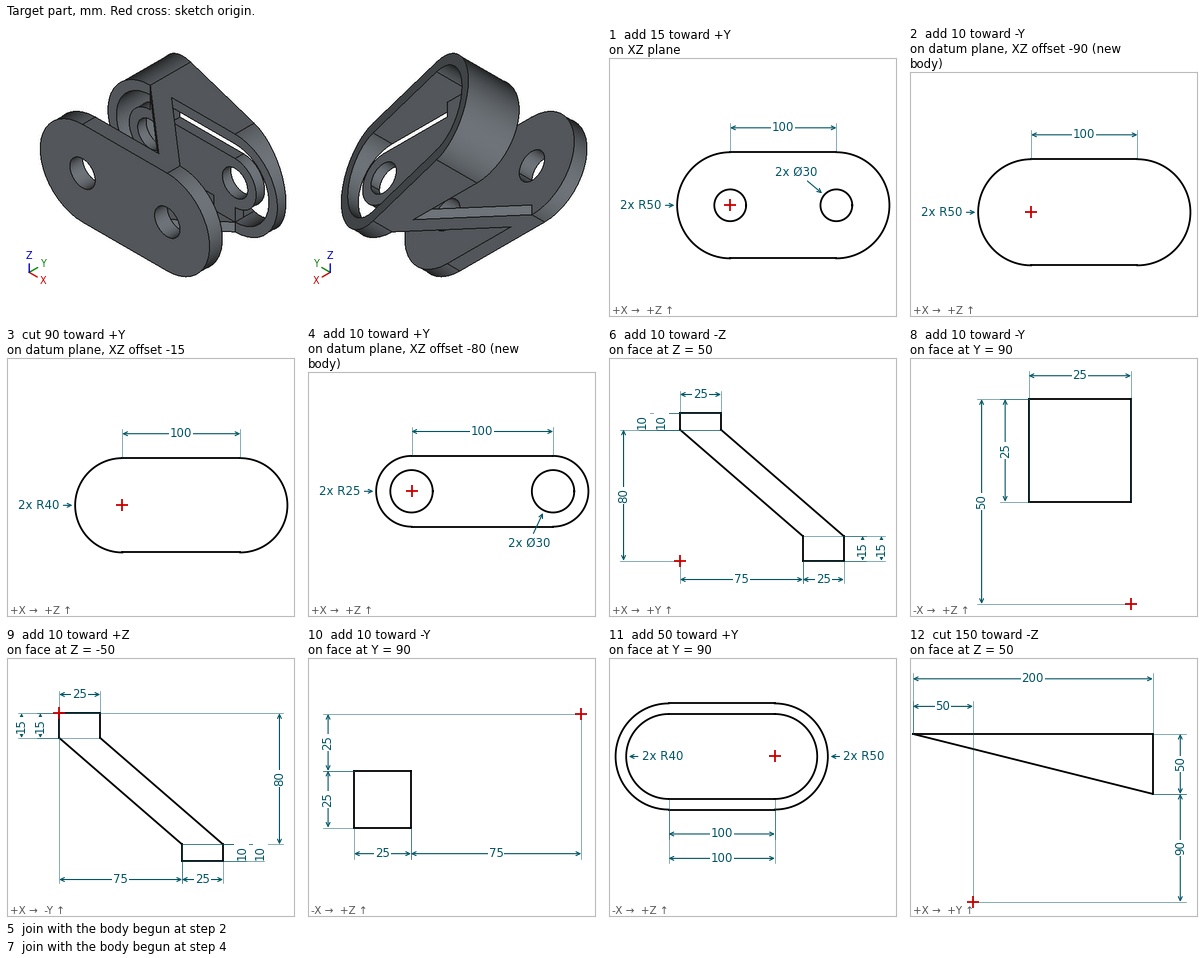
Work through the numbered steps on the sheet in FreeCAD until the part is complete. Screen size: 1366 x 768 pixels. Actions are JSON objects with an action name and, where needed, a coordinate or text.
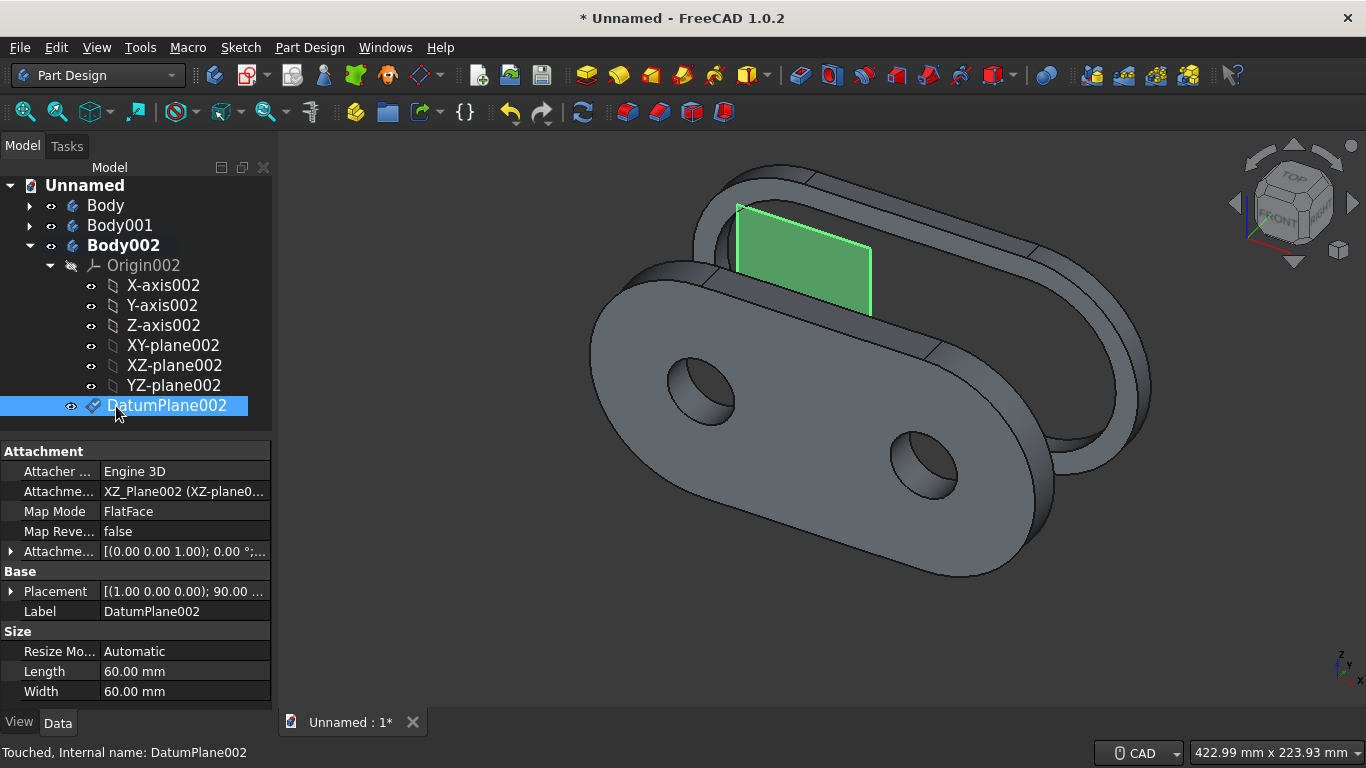
{"action": "left_click", "coordinate": [248, 76]}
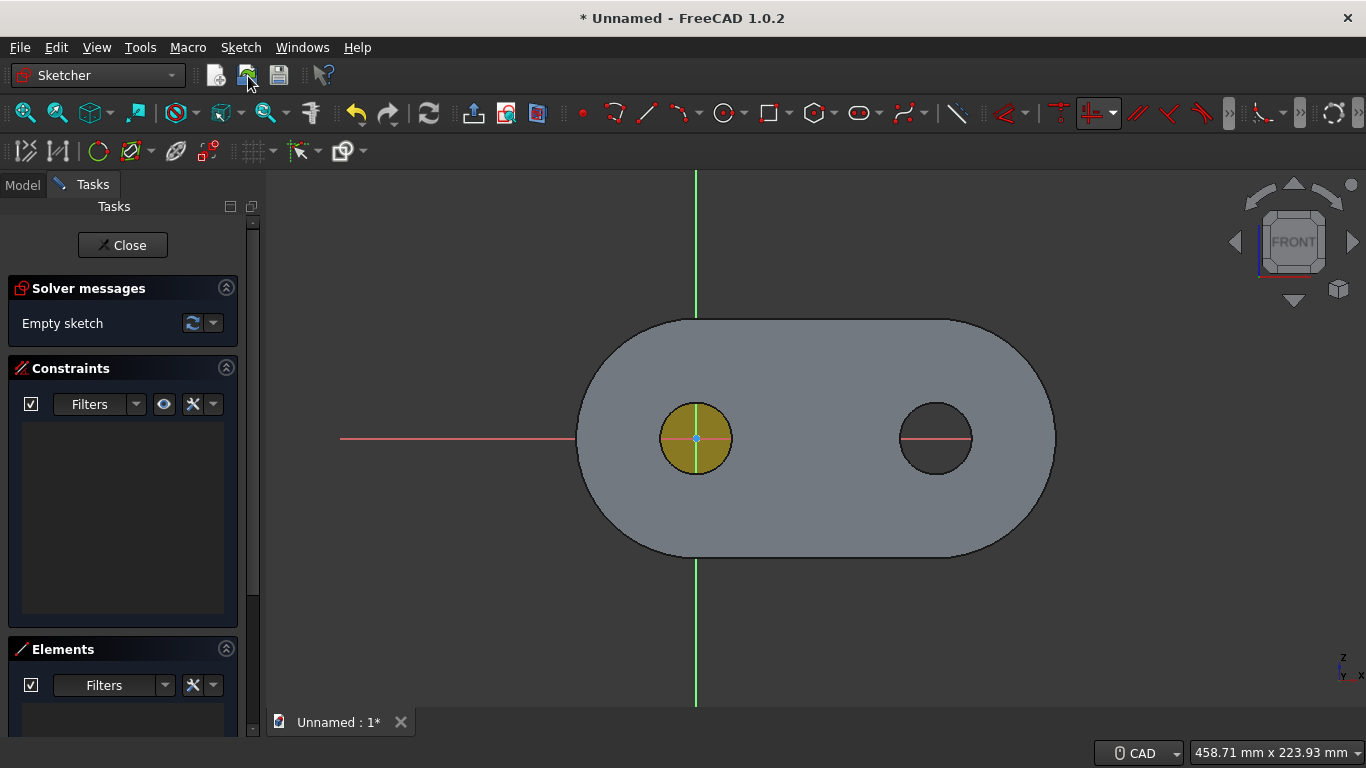
{"action": "scroll", "coordinate": [899, 439], "scroll_direction": "up", "scroll_amount": 3}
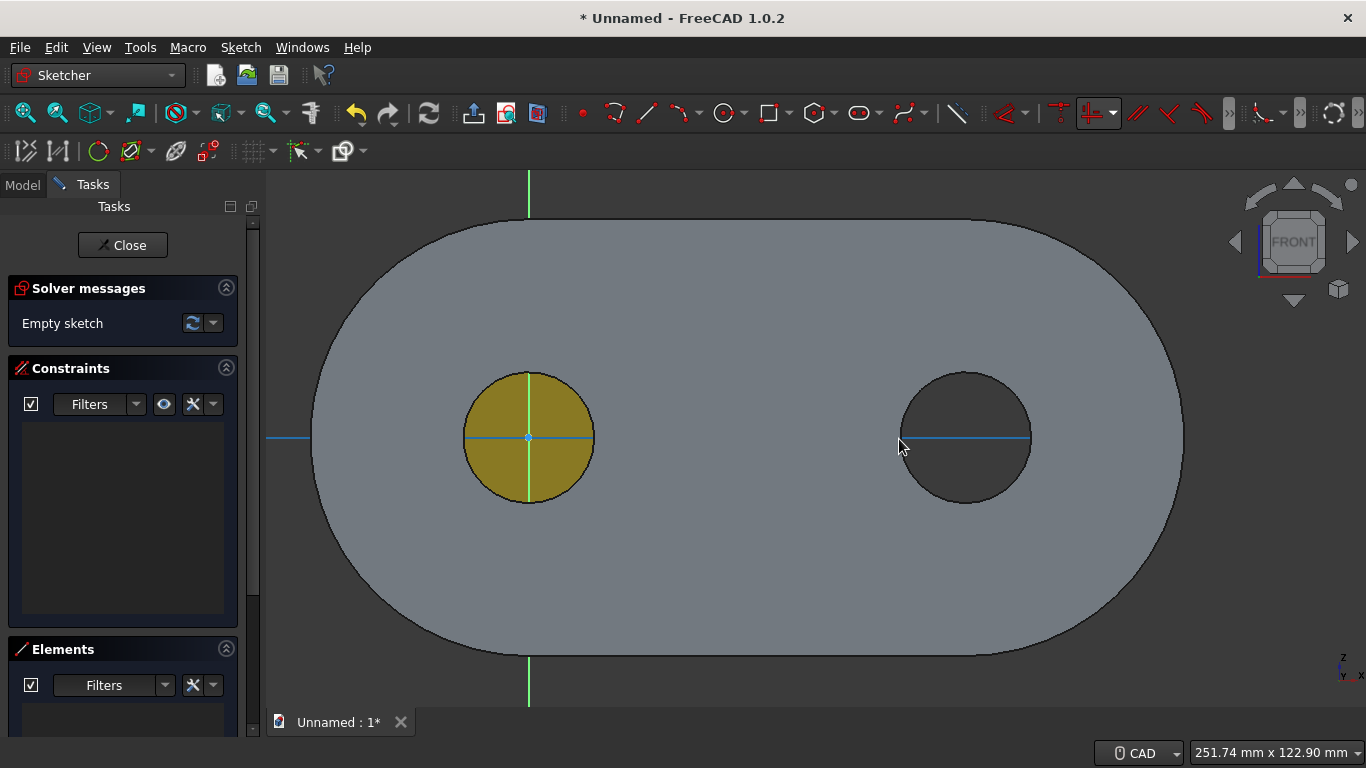
{"action": "left_click", "coordinate": [860, 114]}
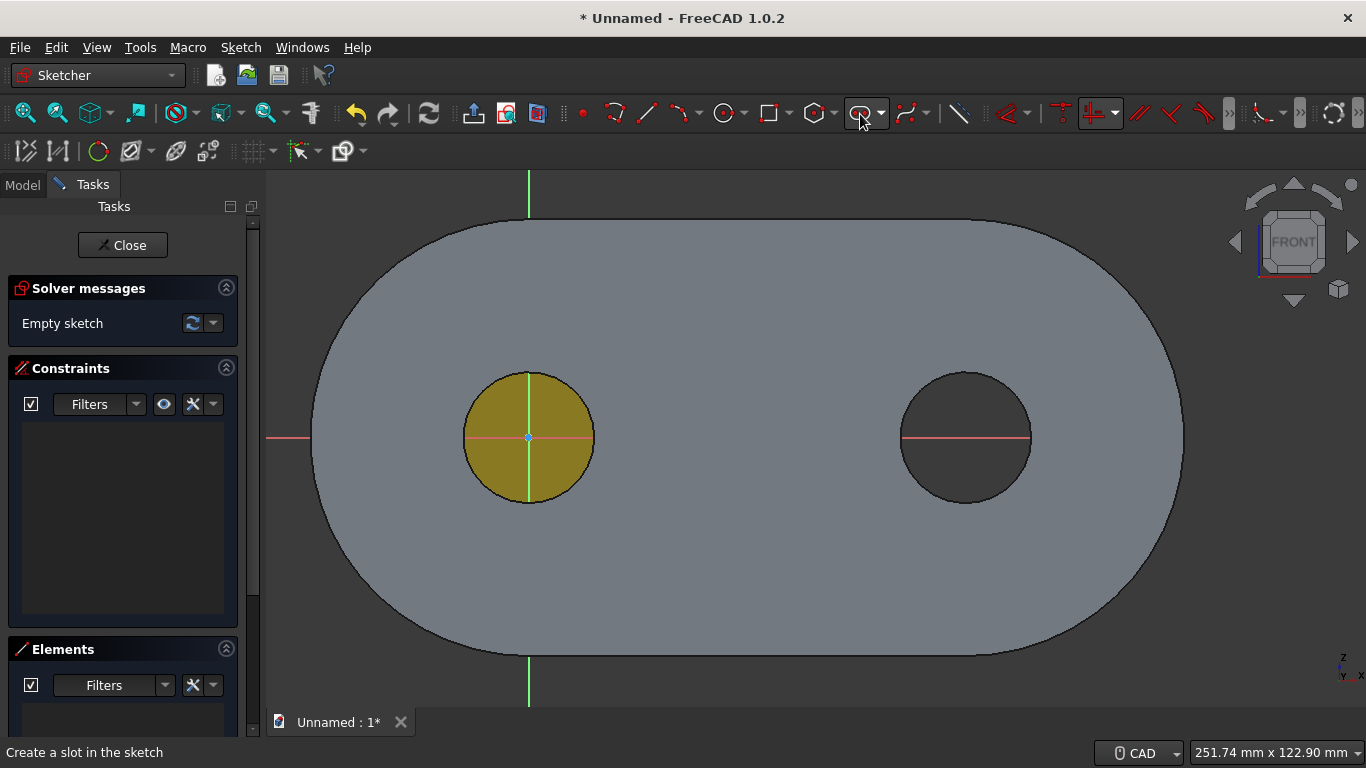
{"action": "left_click", "coordinate": [529, 438]}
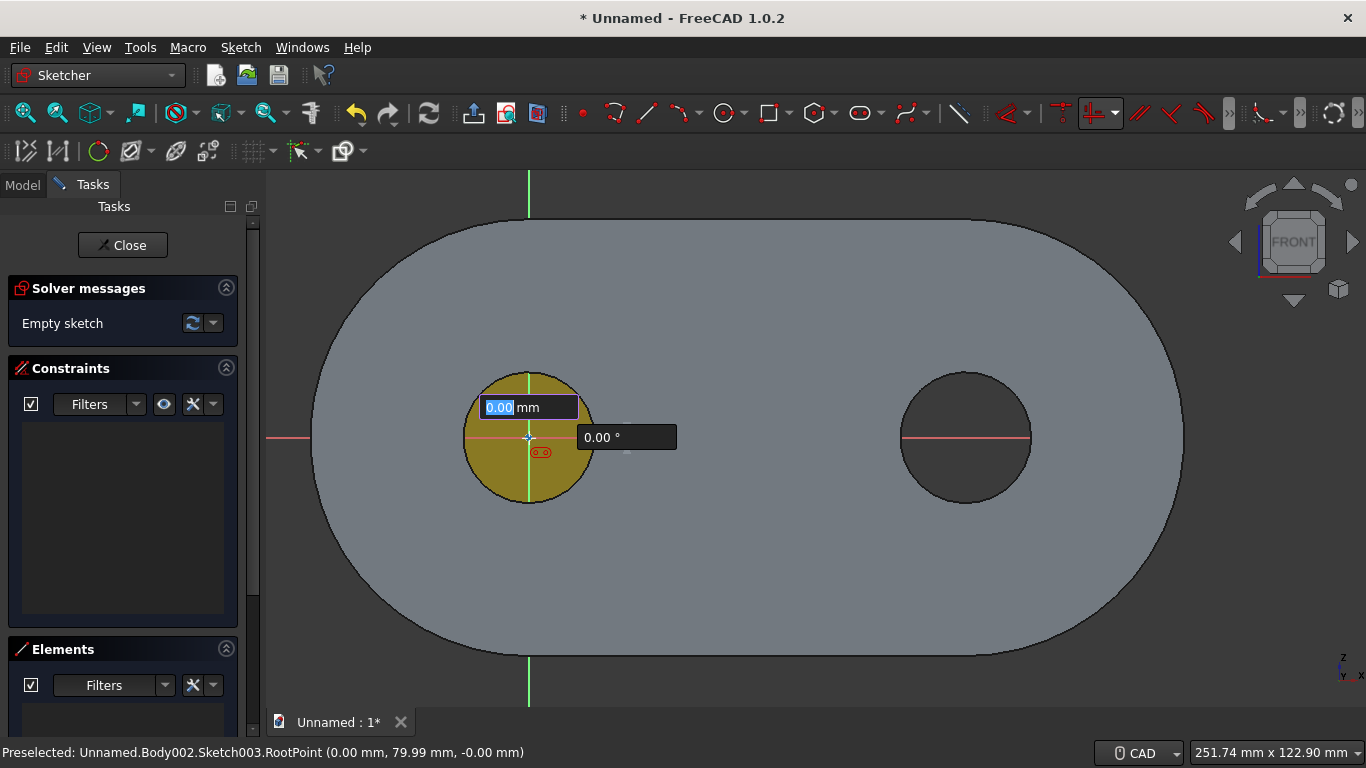
{"action": "left_click", "coordinate": [966, 429]}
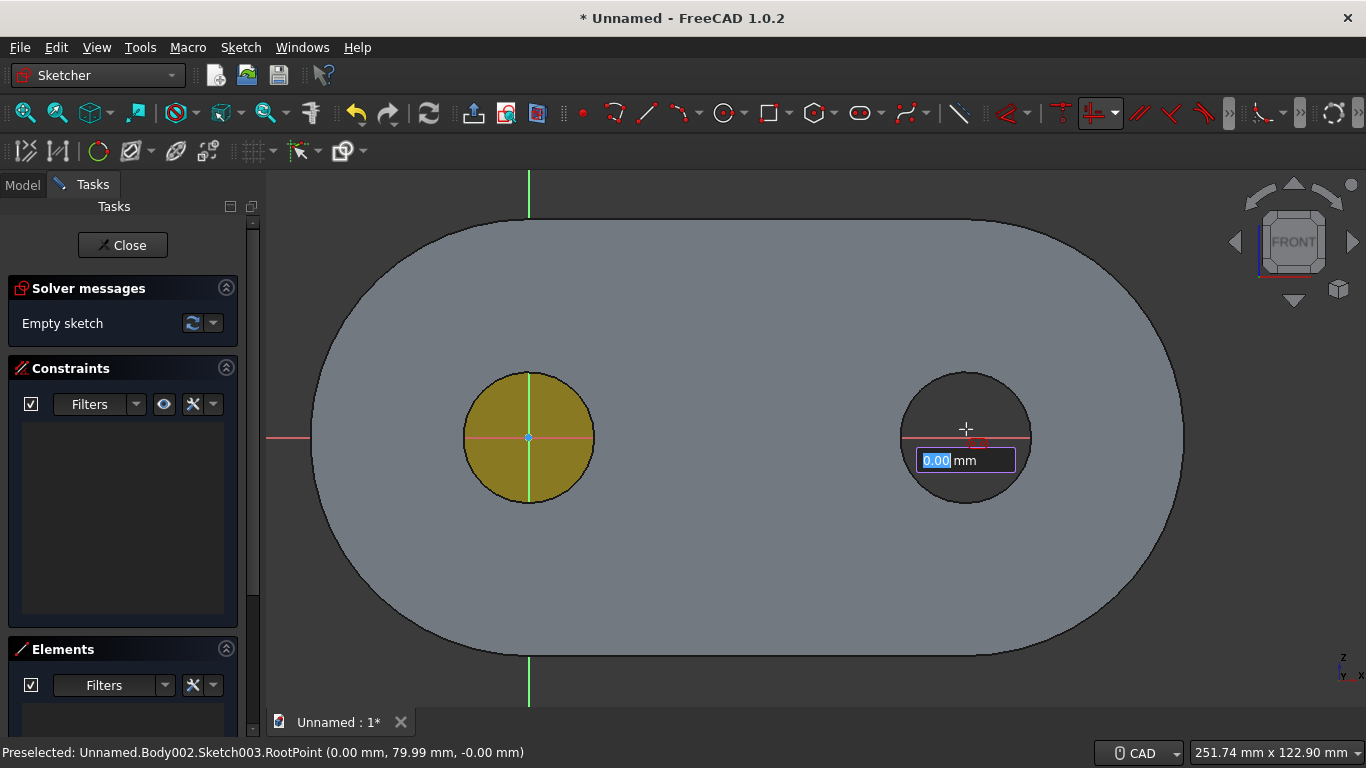
{"action": "left_click", "coordinate": [747, 547]}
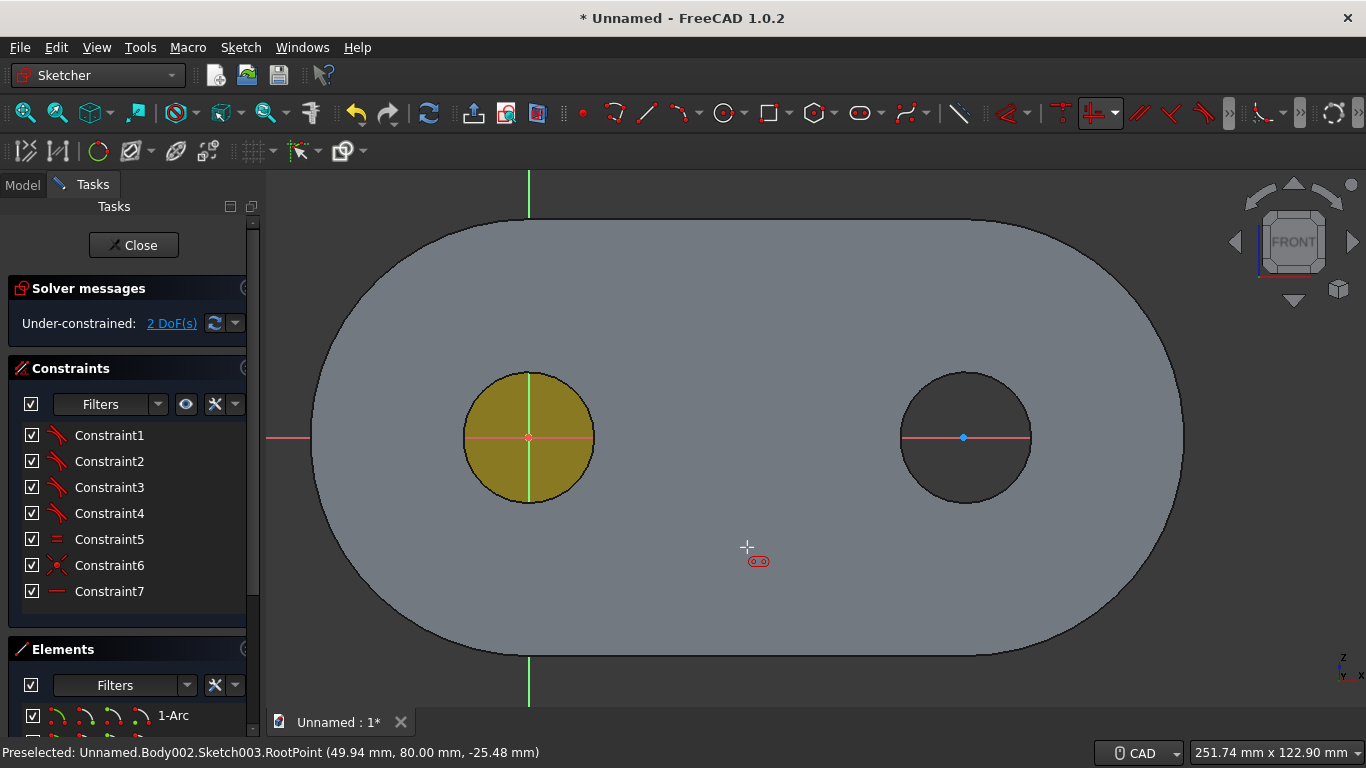
{"action": "left_click", "coordinate": [724, 114]}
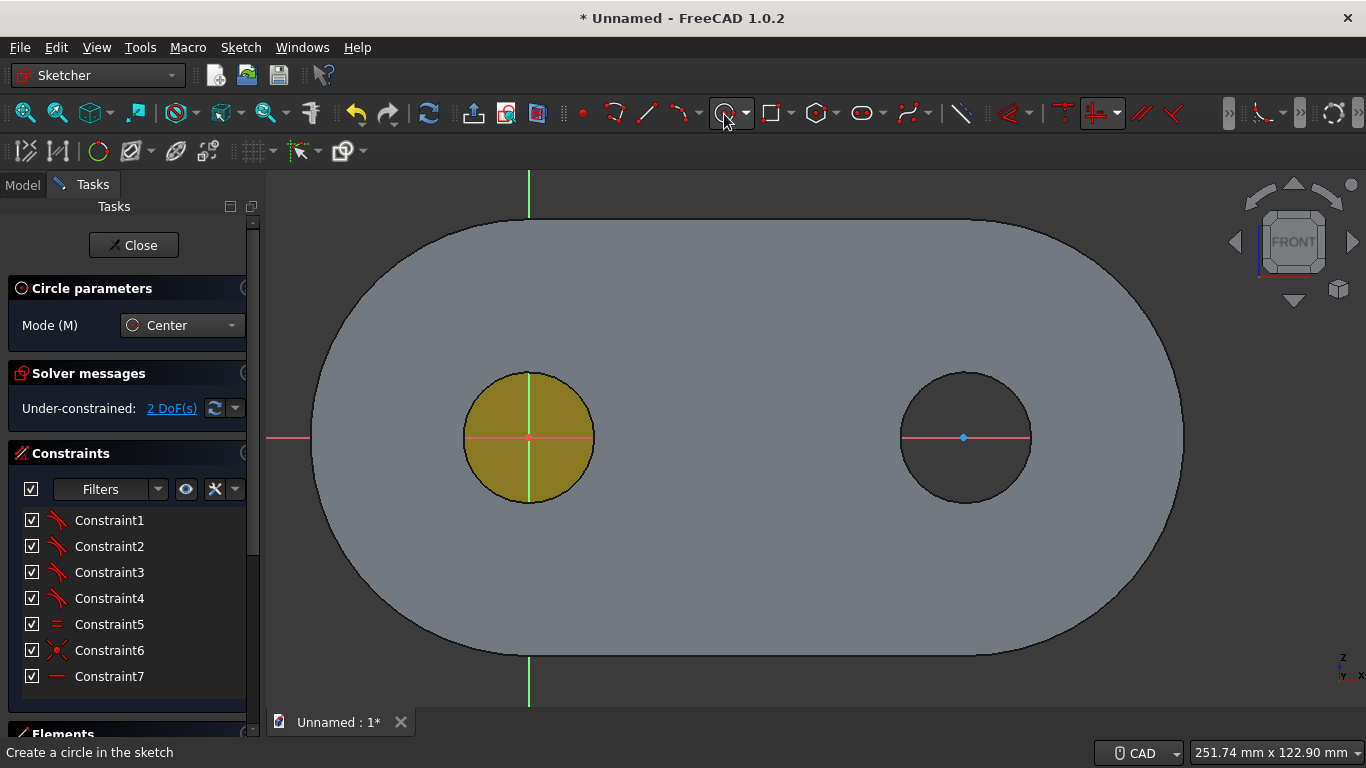
{"action": "left_click", "coordinate": [964, 438]}
{"action": "left_click", "coordinate": [1012, 391]}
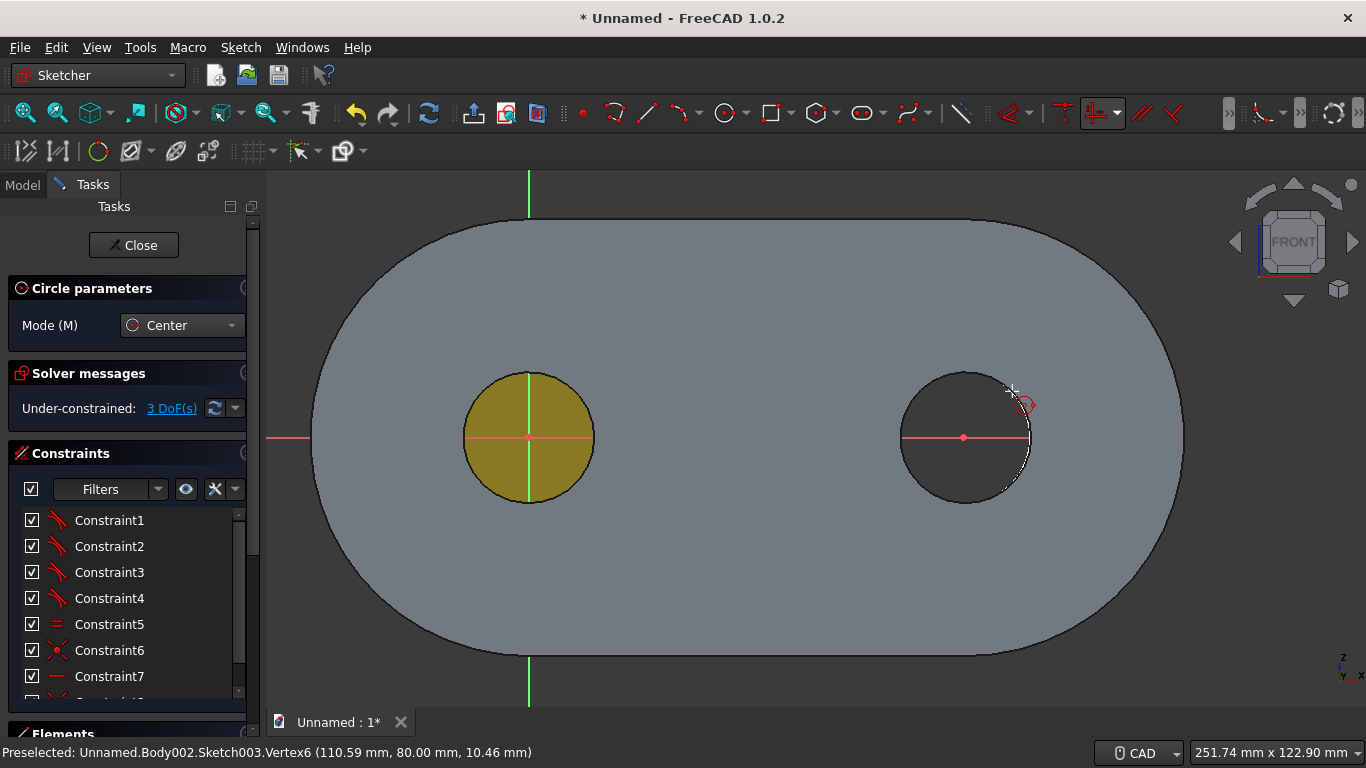
{"action": "left_click", "coordinate": [529, 438]}
{"action": "left_click", "coordinate": [575, 391]}
{"action": "key", "text": "Escape"}